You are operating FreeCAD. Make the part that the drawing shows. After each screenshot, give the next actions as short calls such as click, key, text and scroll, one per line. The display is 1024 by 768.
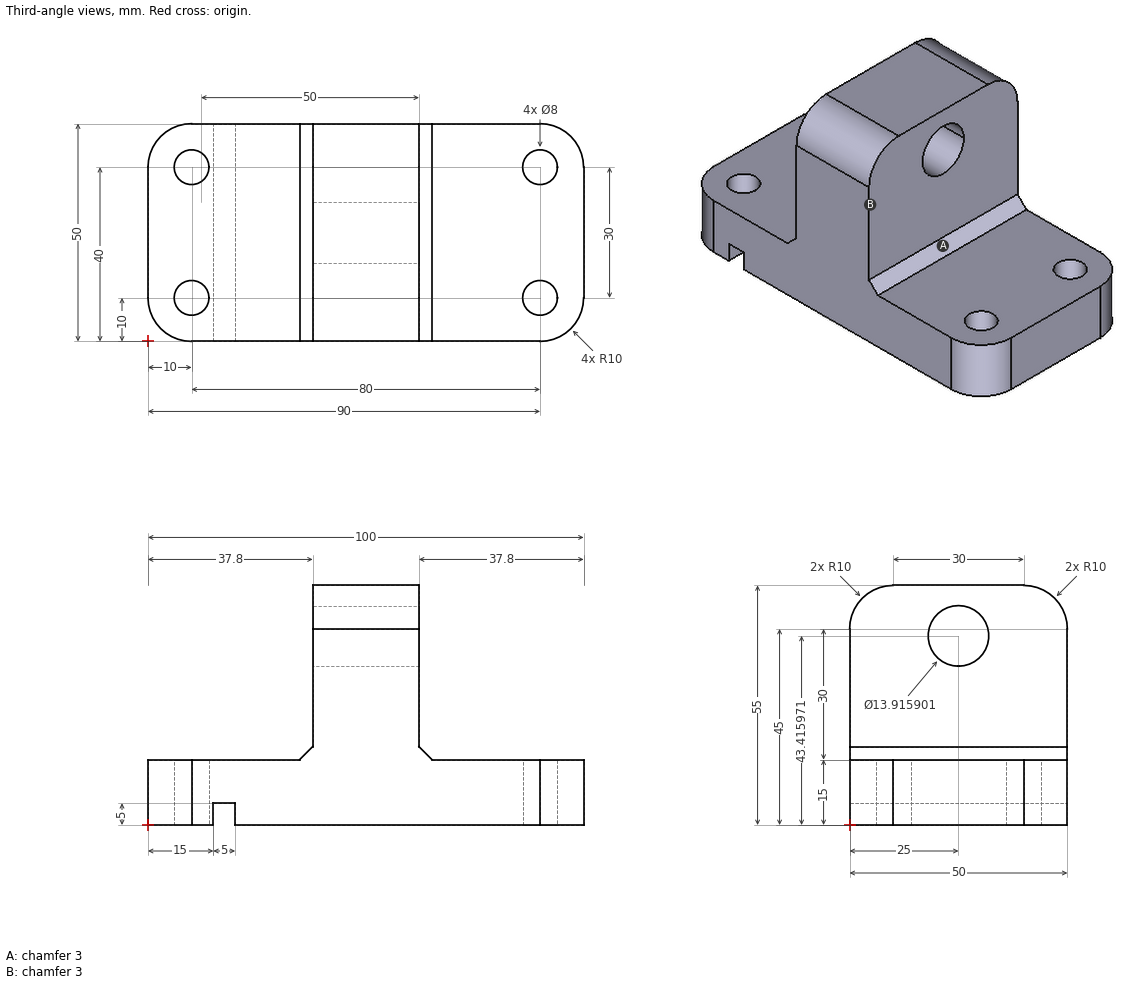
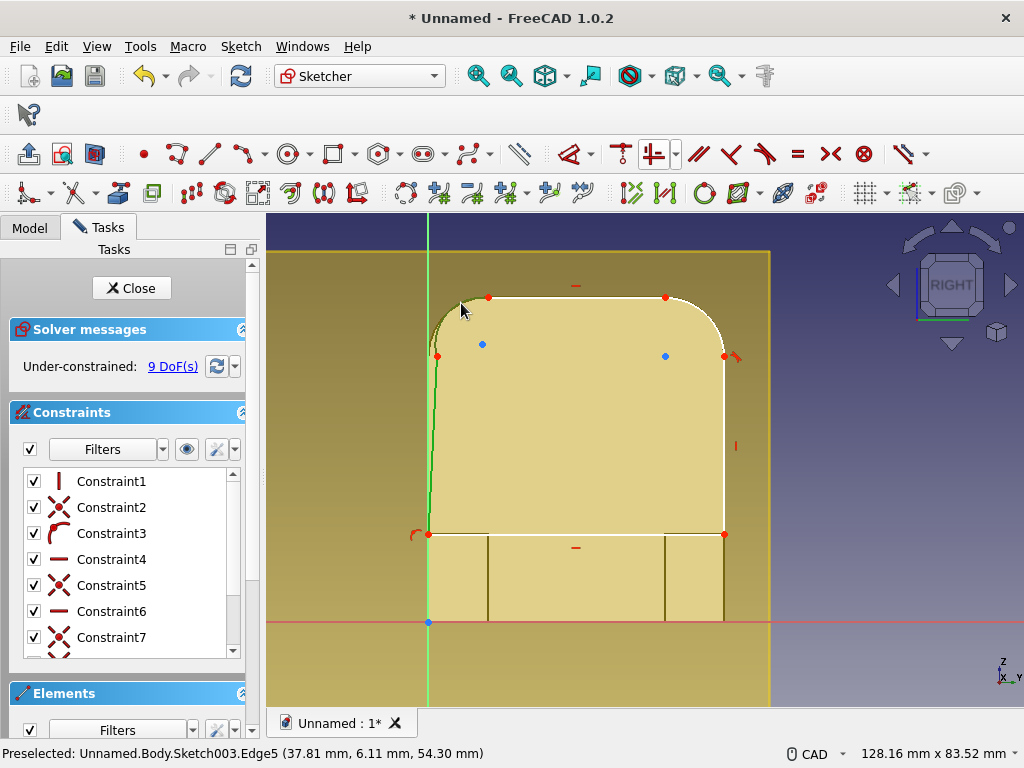
click(765, 154)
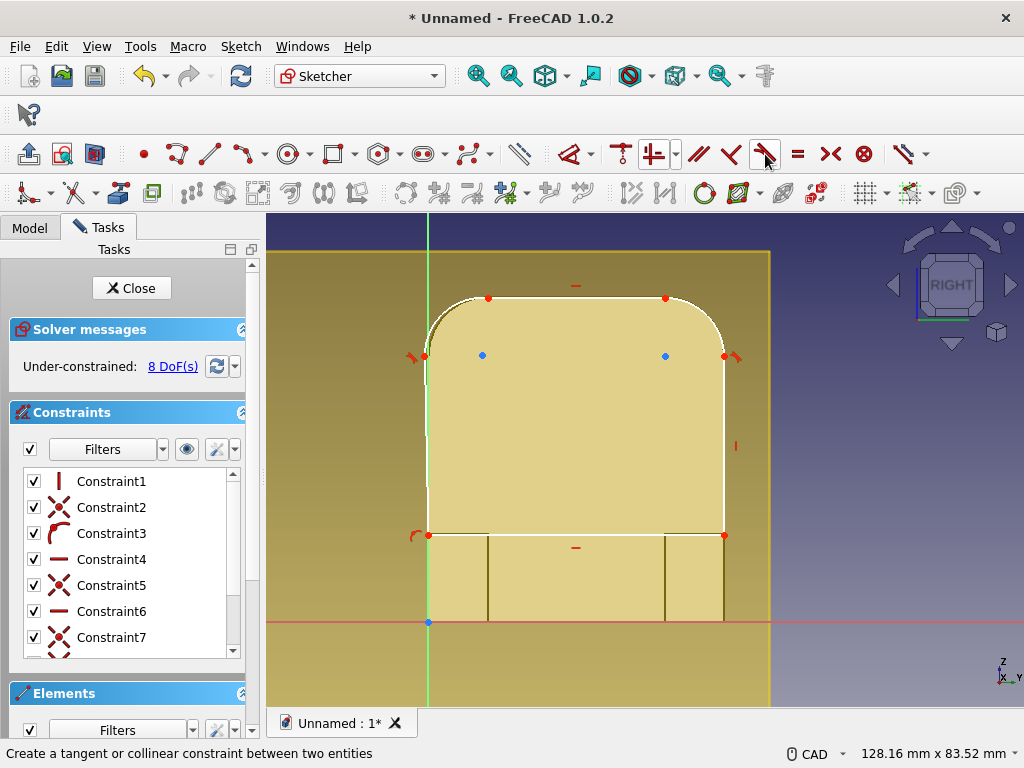
click(541, 298)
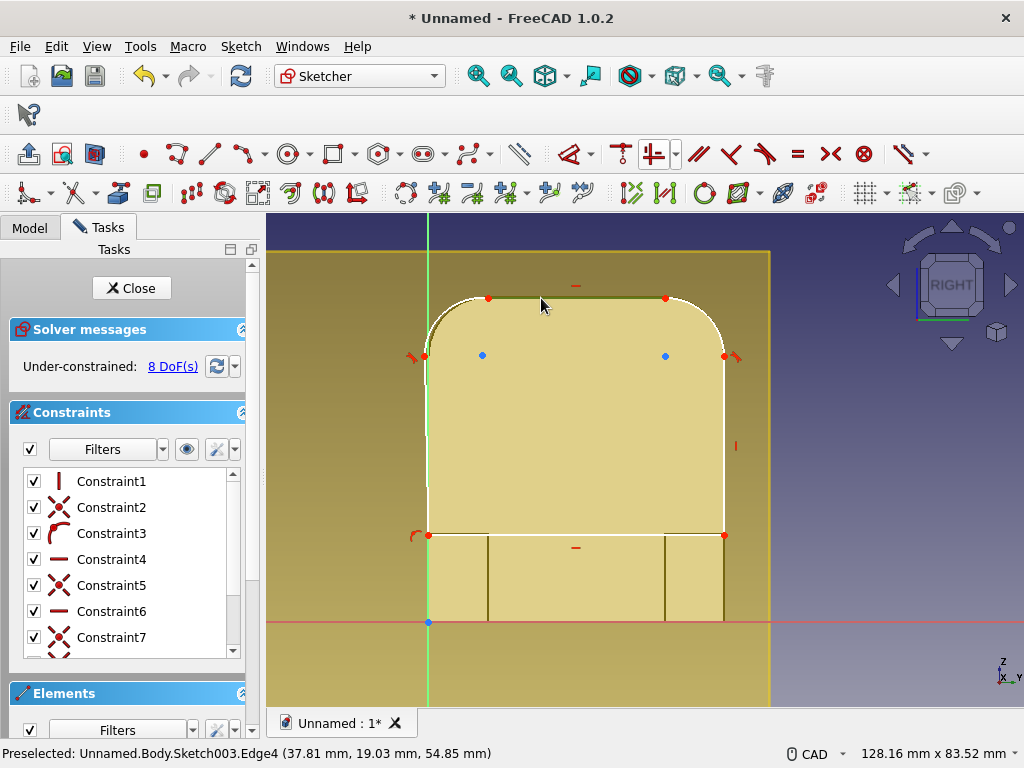
click(460, 303)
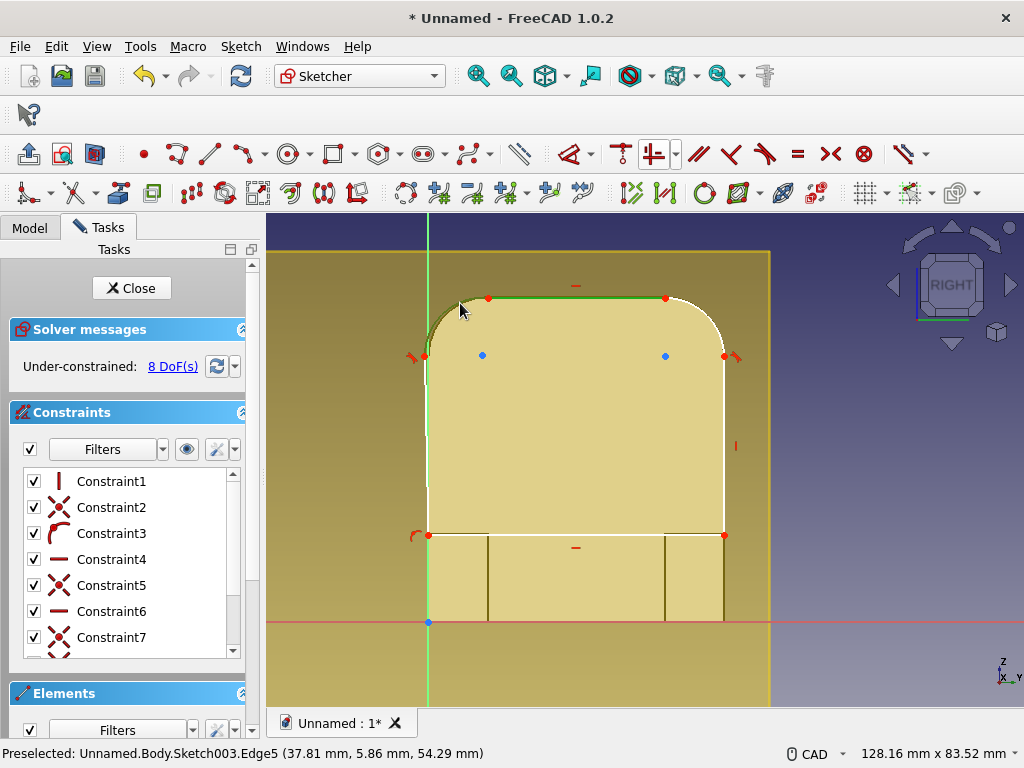
click(765, 154)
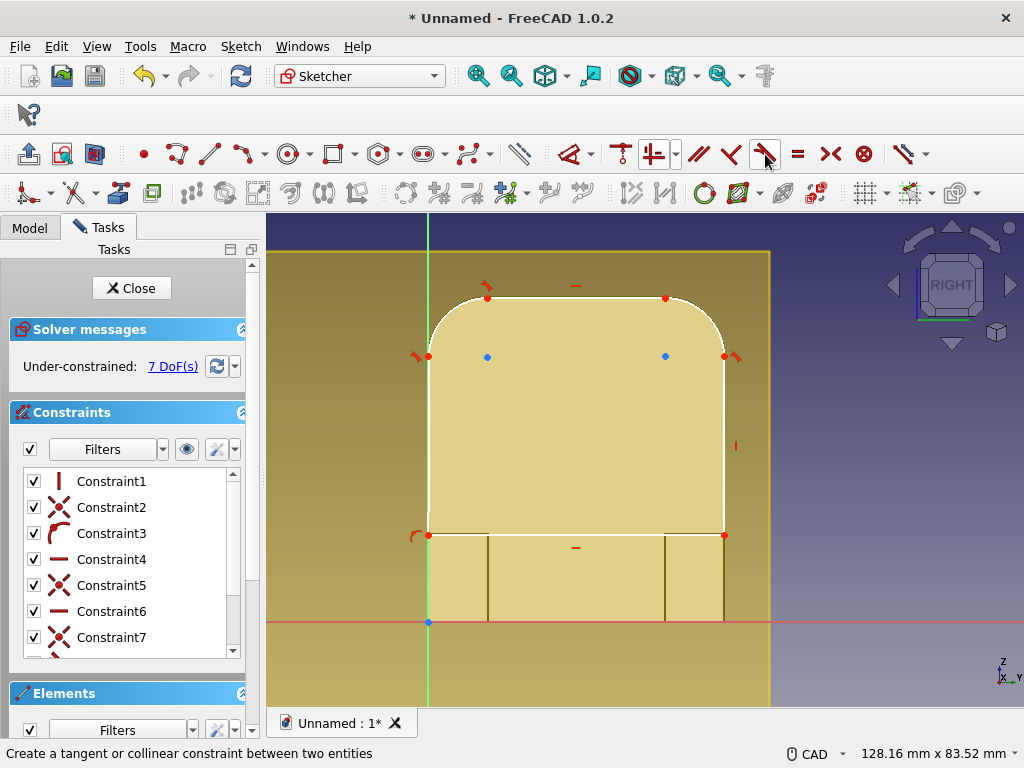
click(541, 298)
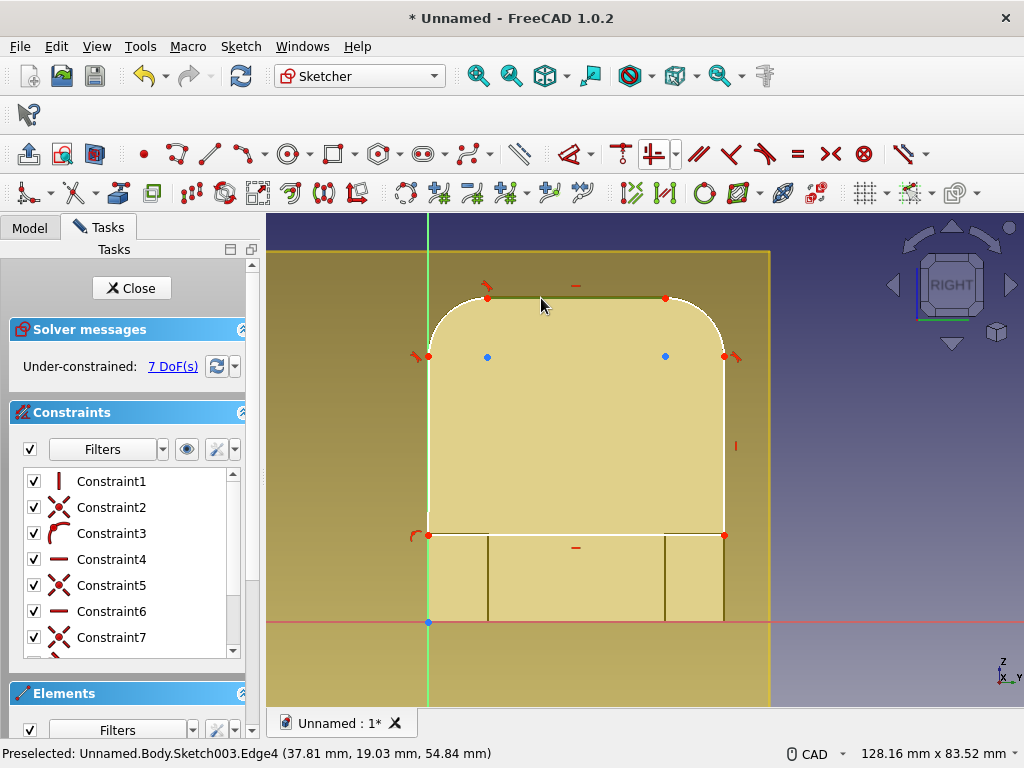
click(718, 330)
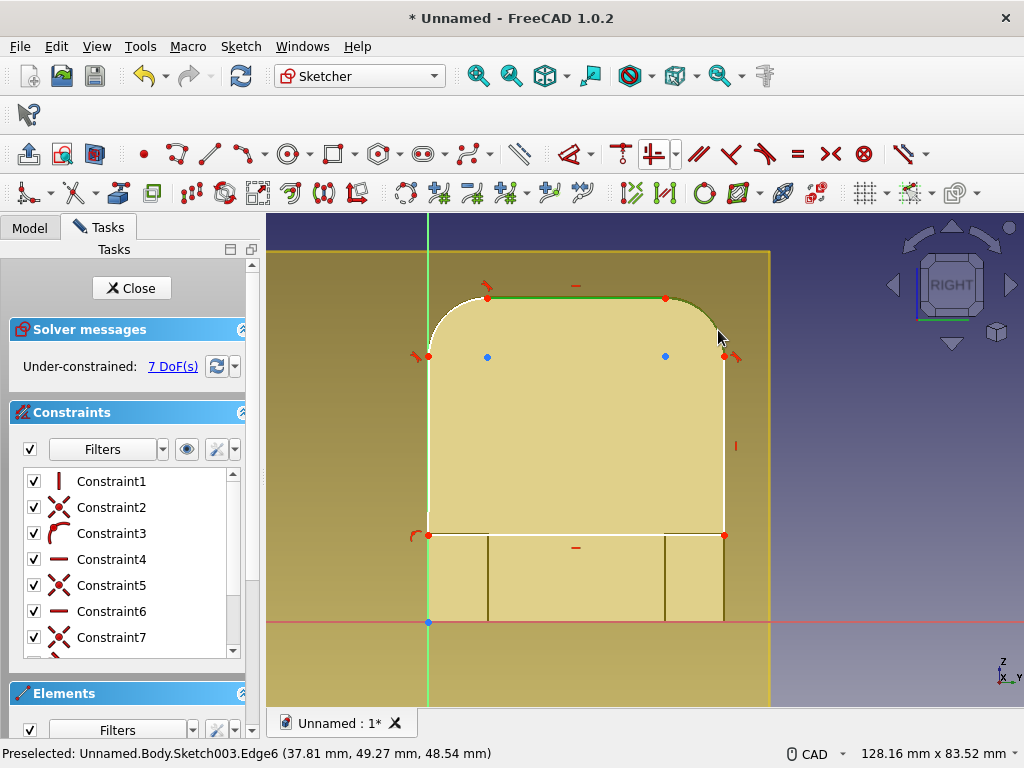
click(765, 154)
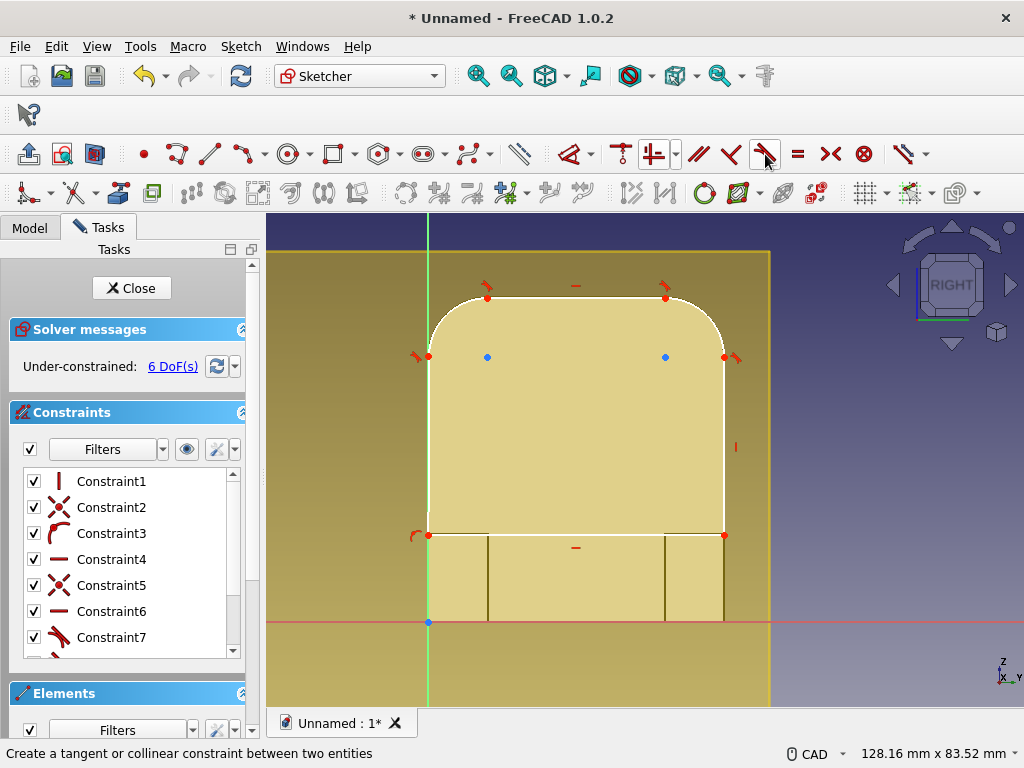
click(429, 482)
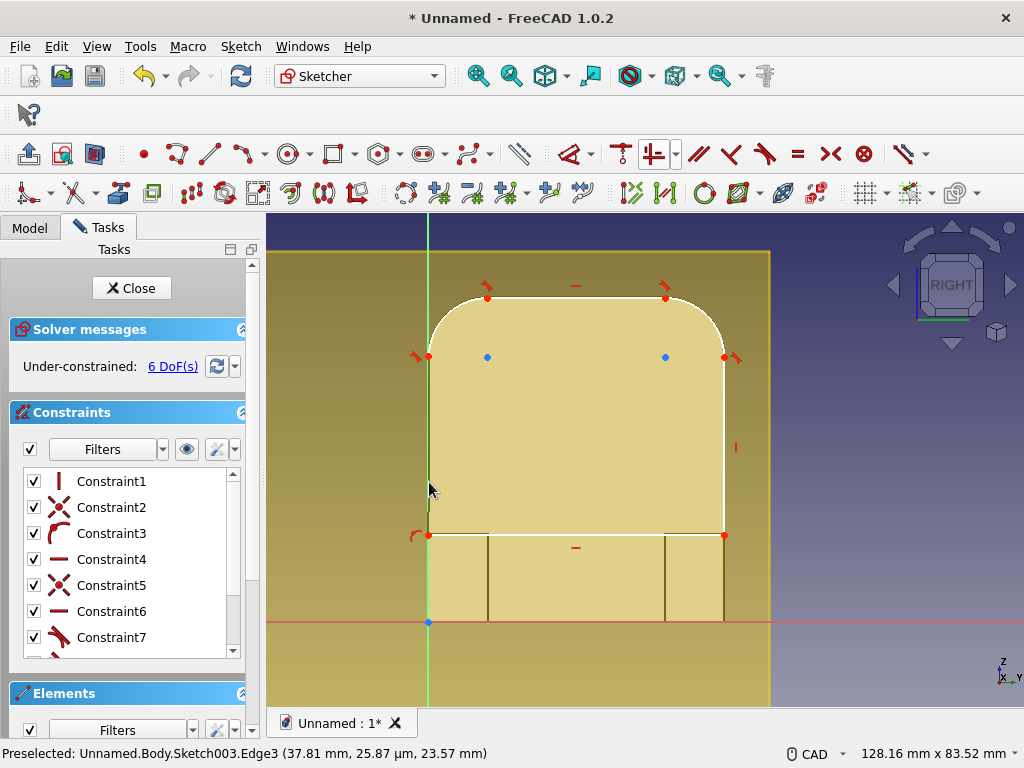
click(676, 154)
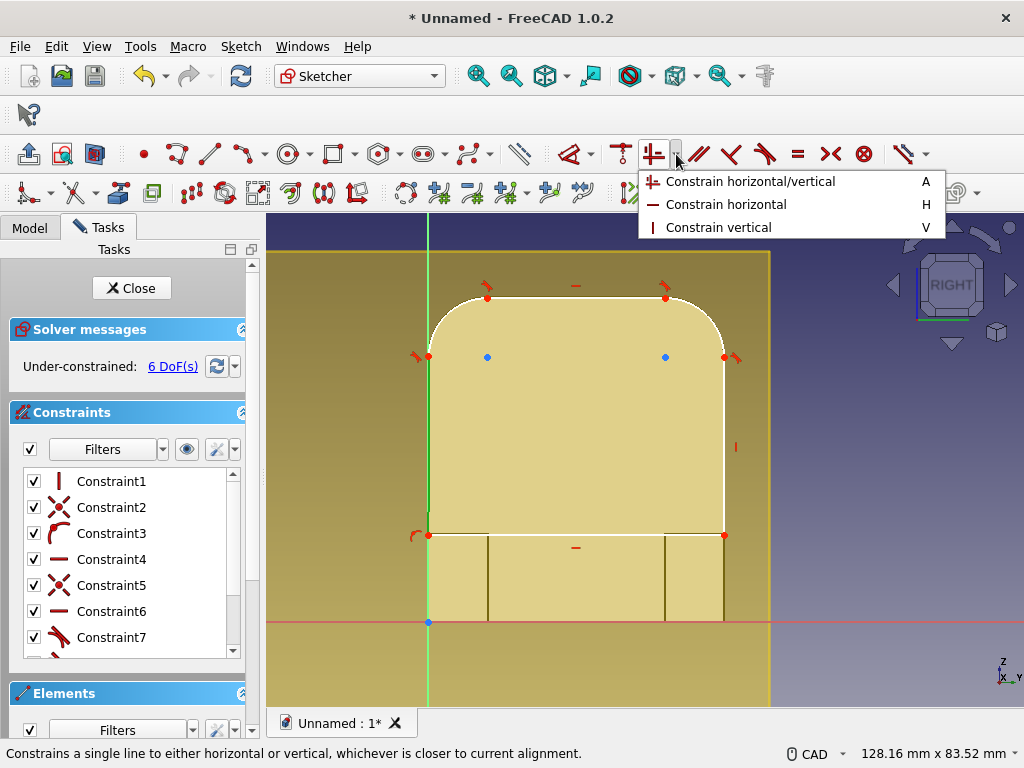
click(792, 228)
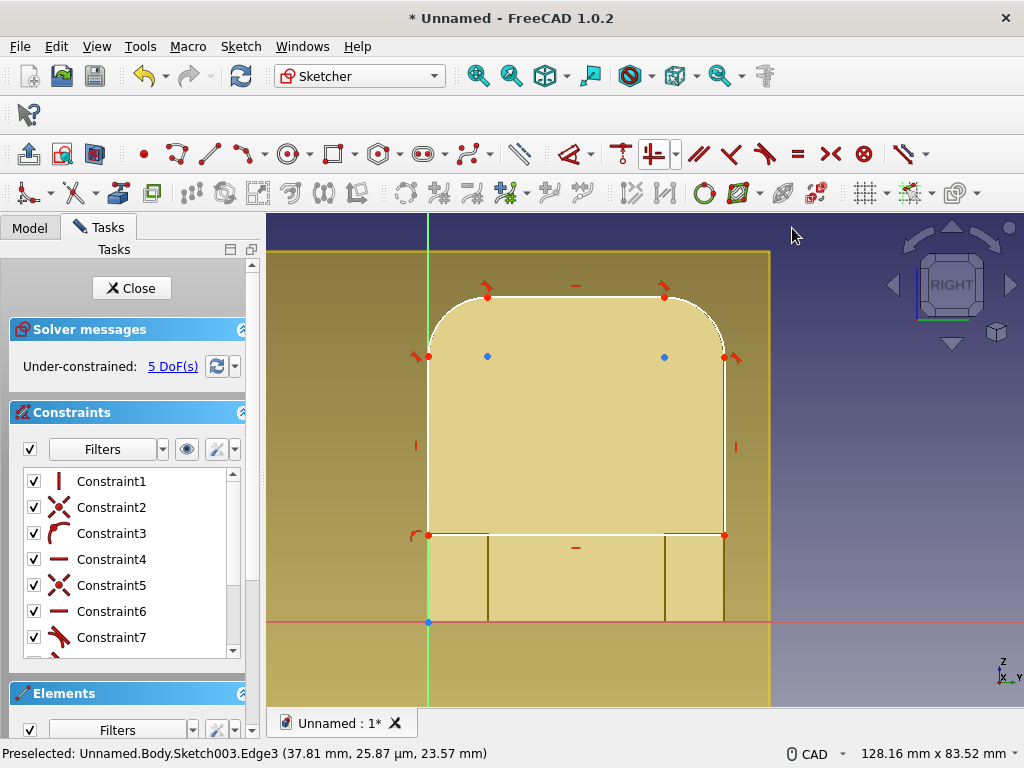
click(461, 304)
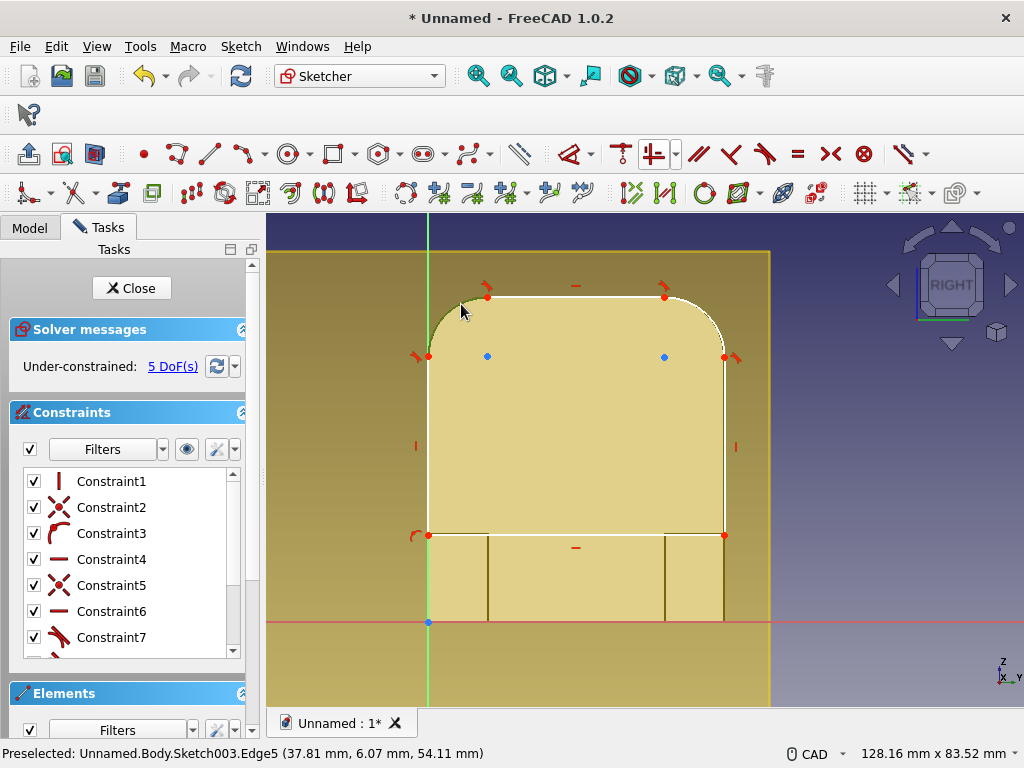
click(718, 330)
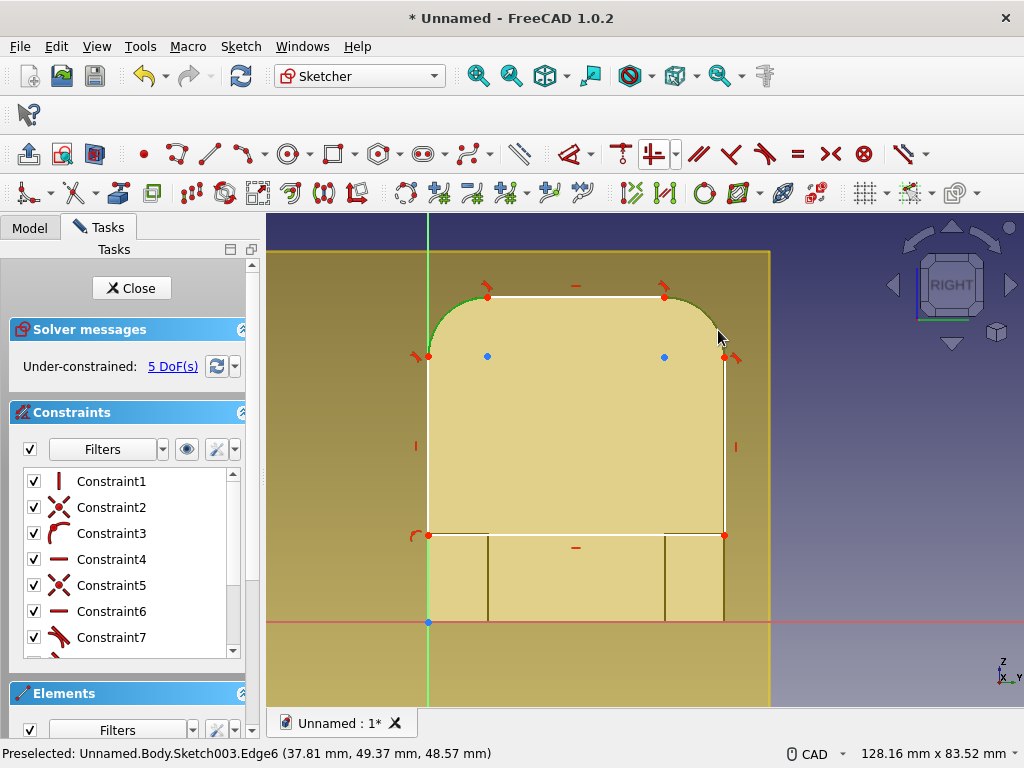
click(798, 154)